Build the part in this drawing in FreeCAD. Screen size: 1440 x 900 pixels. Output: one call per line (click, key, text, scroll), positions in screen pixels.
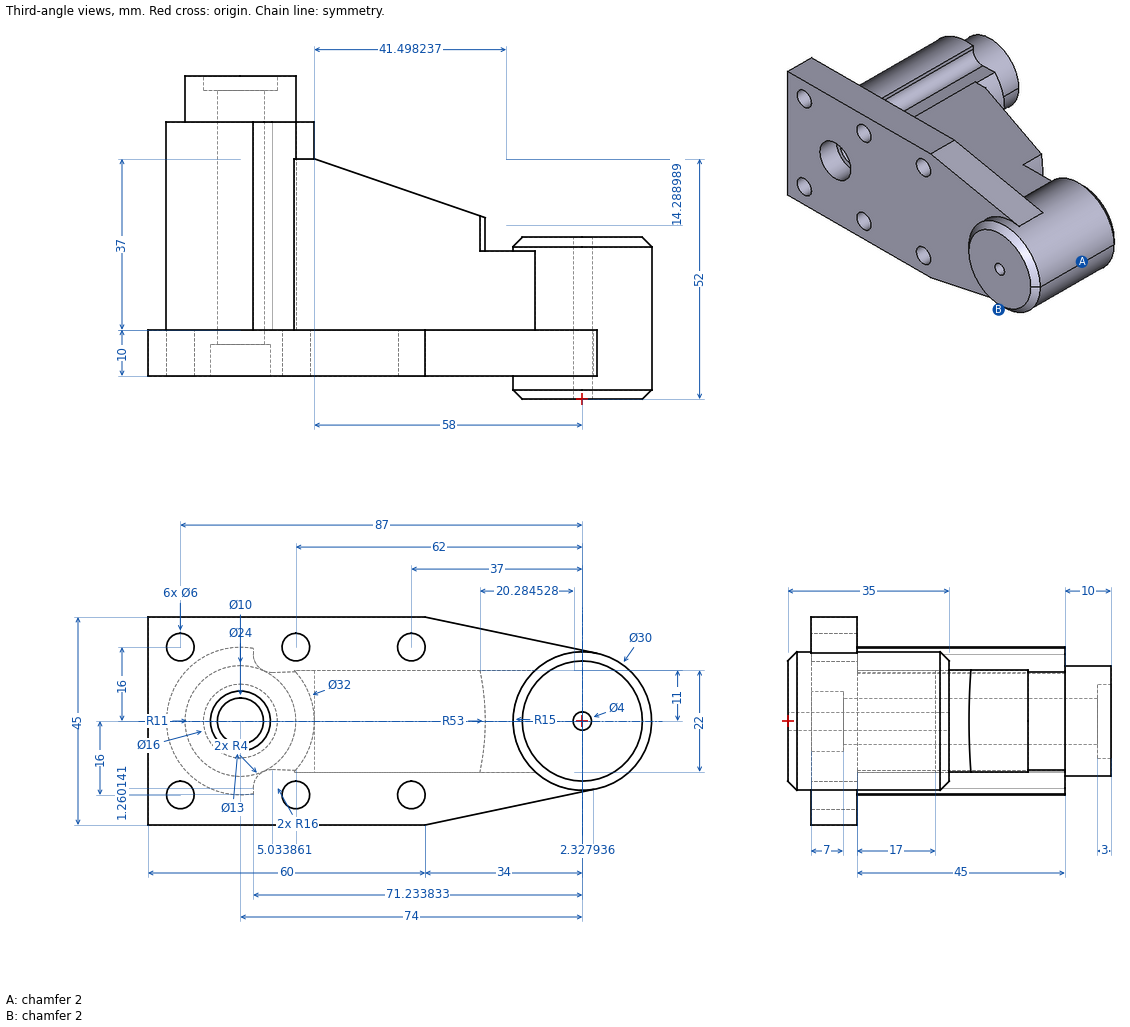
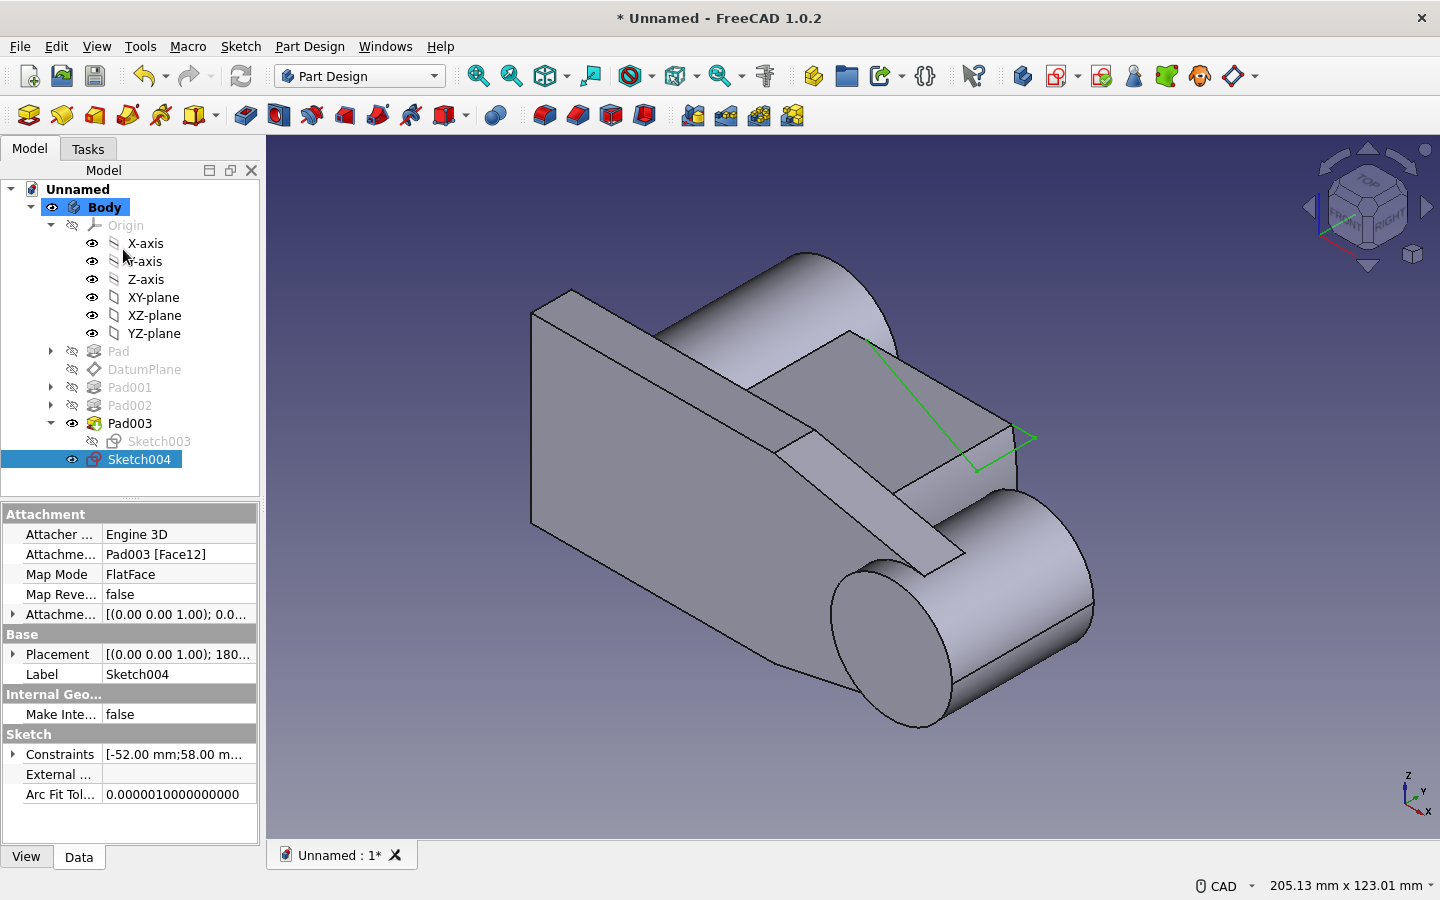
click(246, 116)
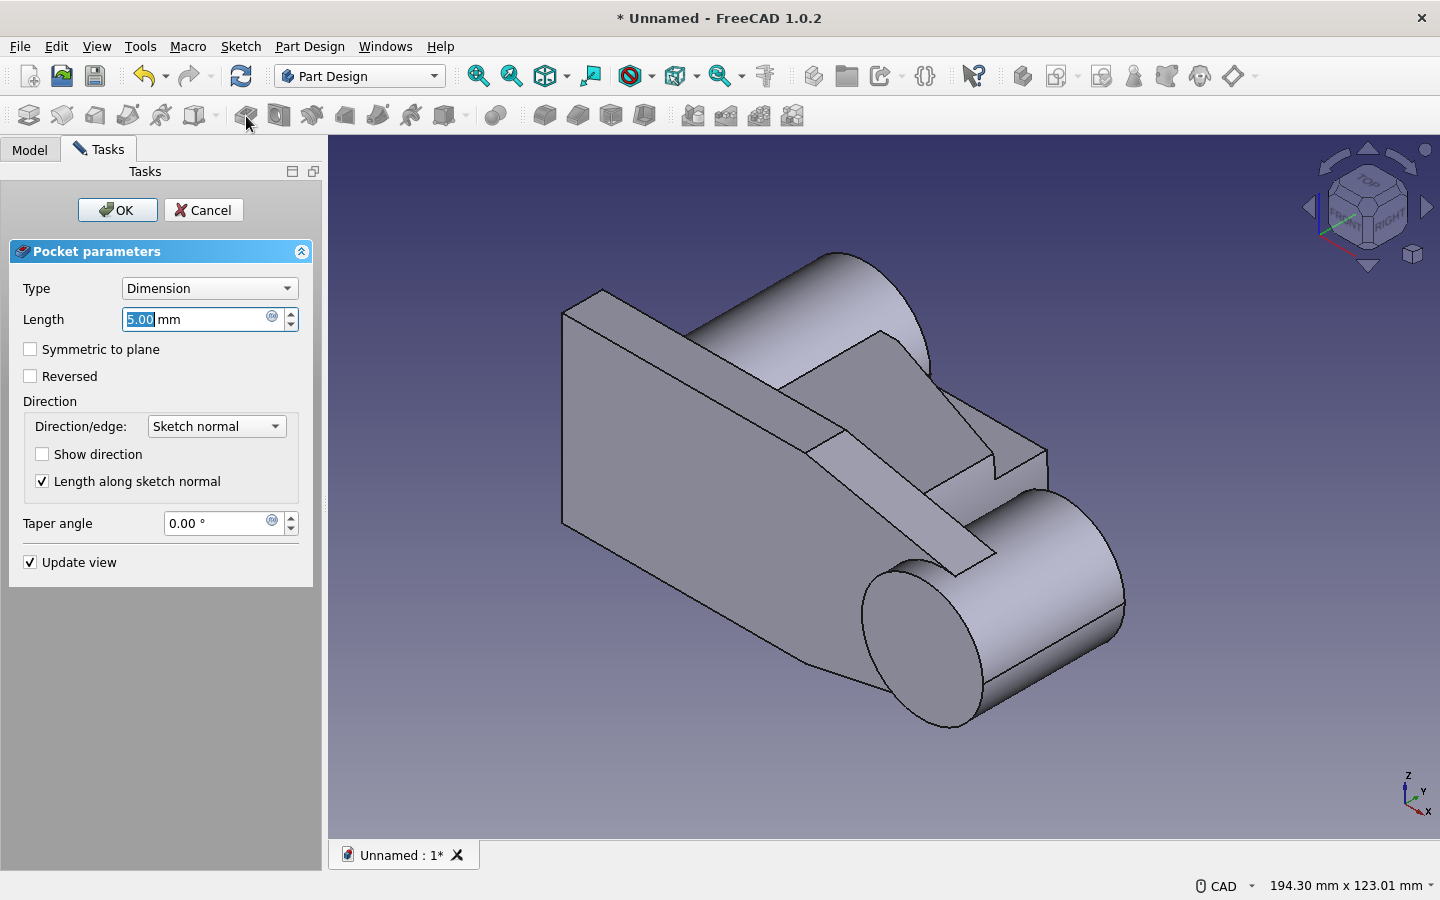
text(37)
key(Tab)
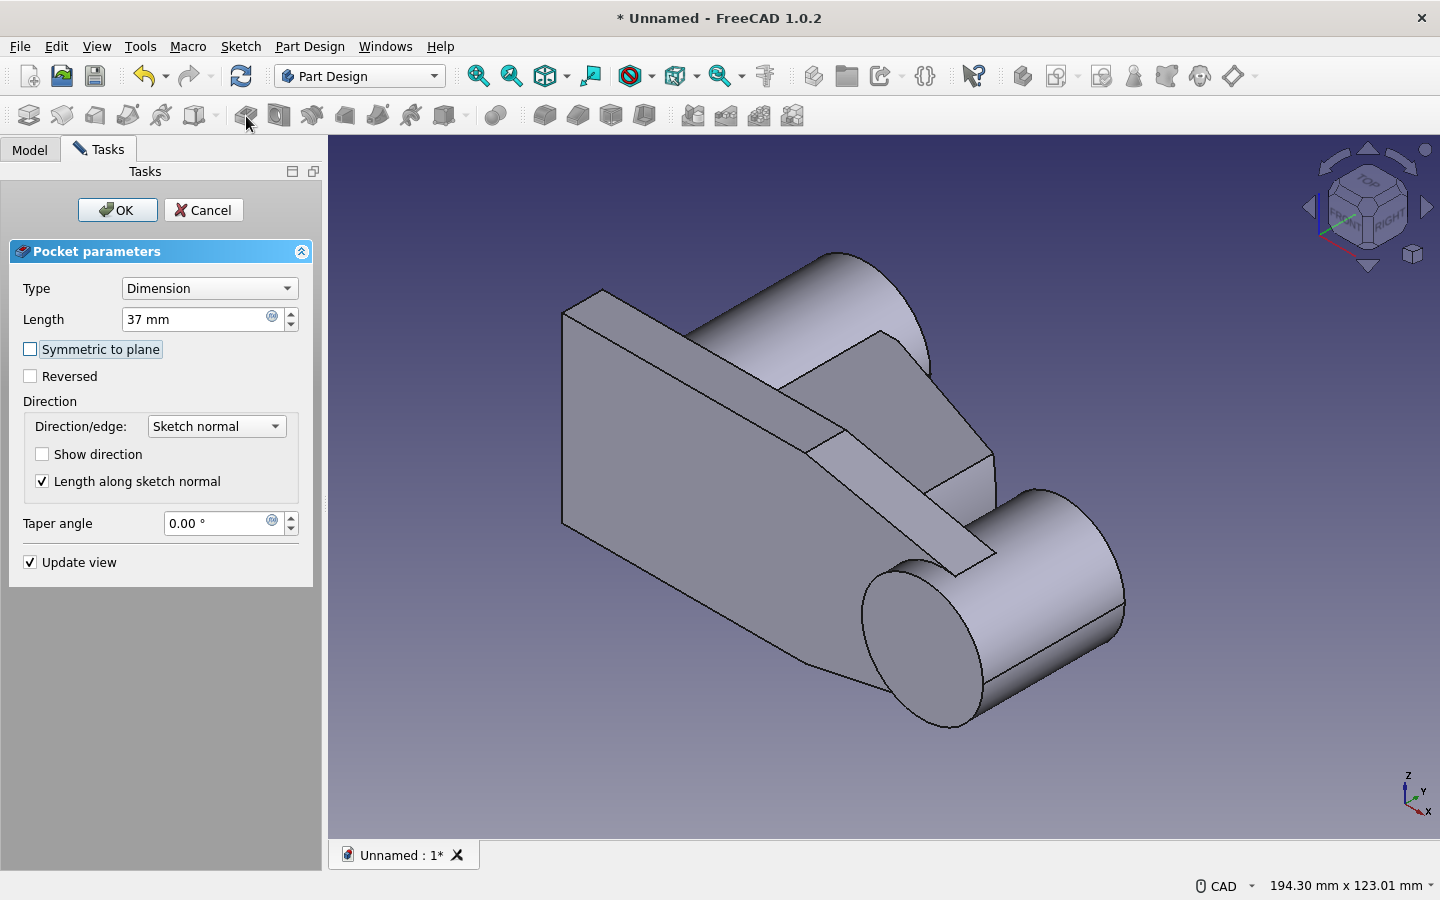
click(118, 210)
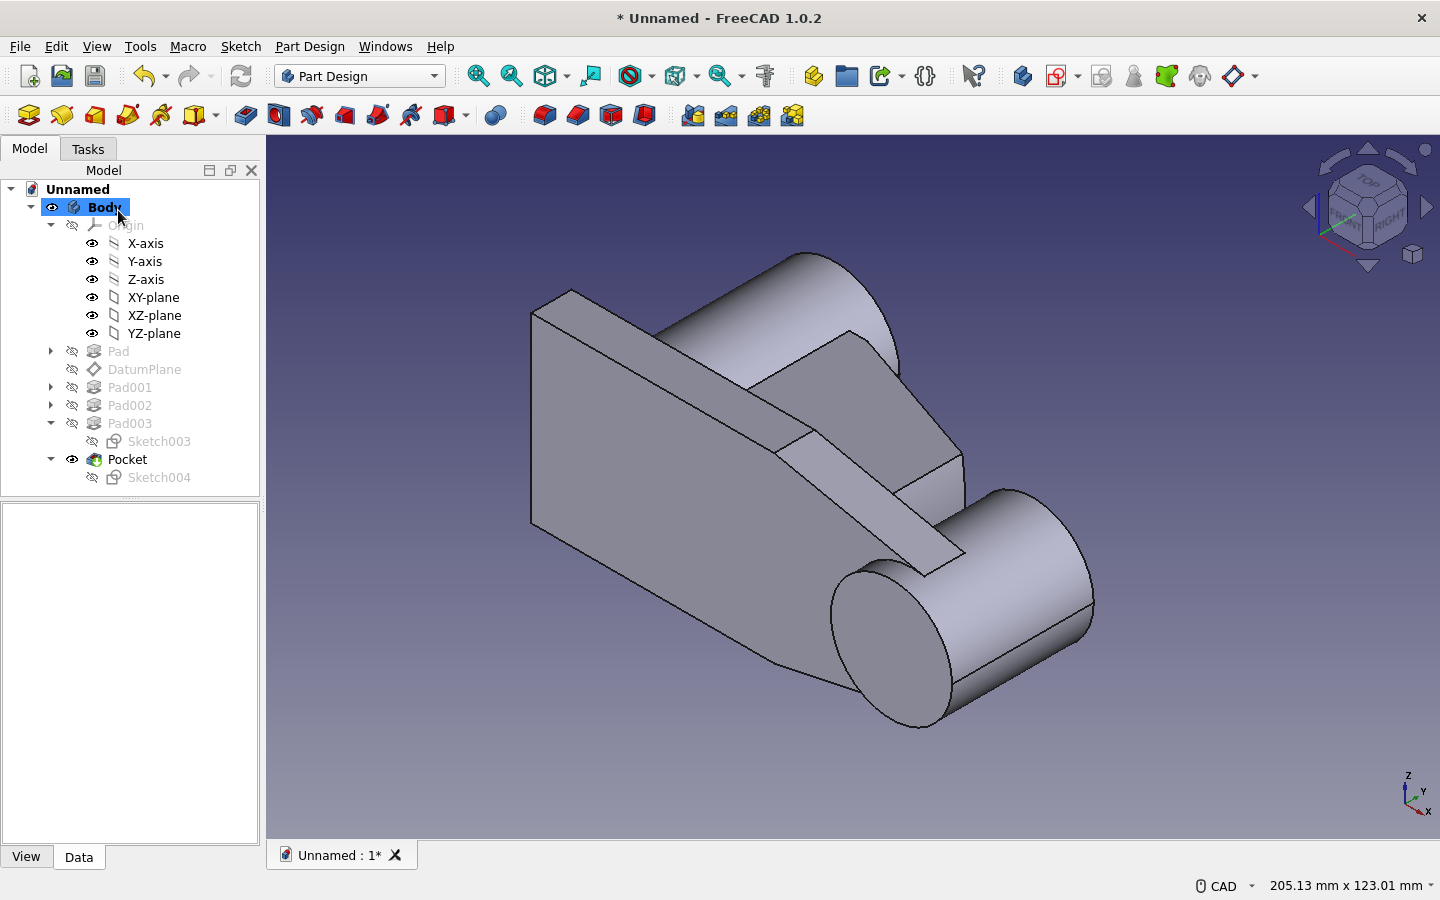
key(4)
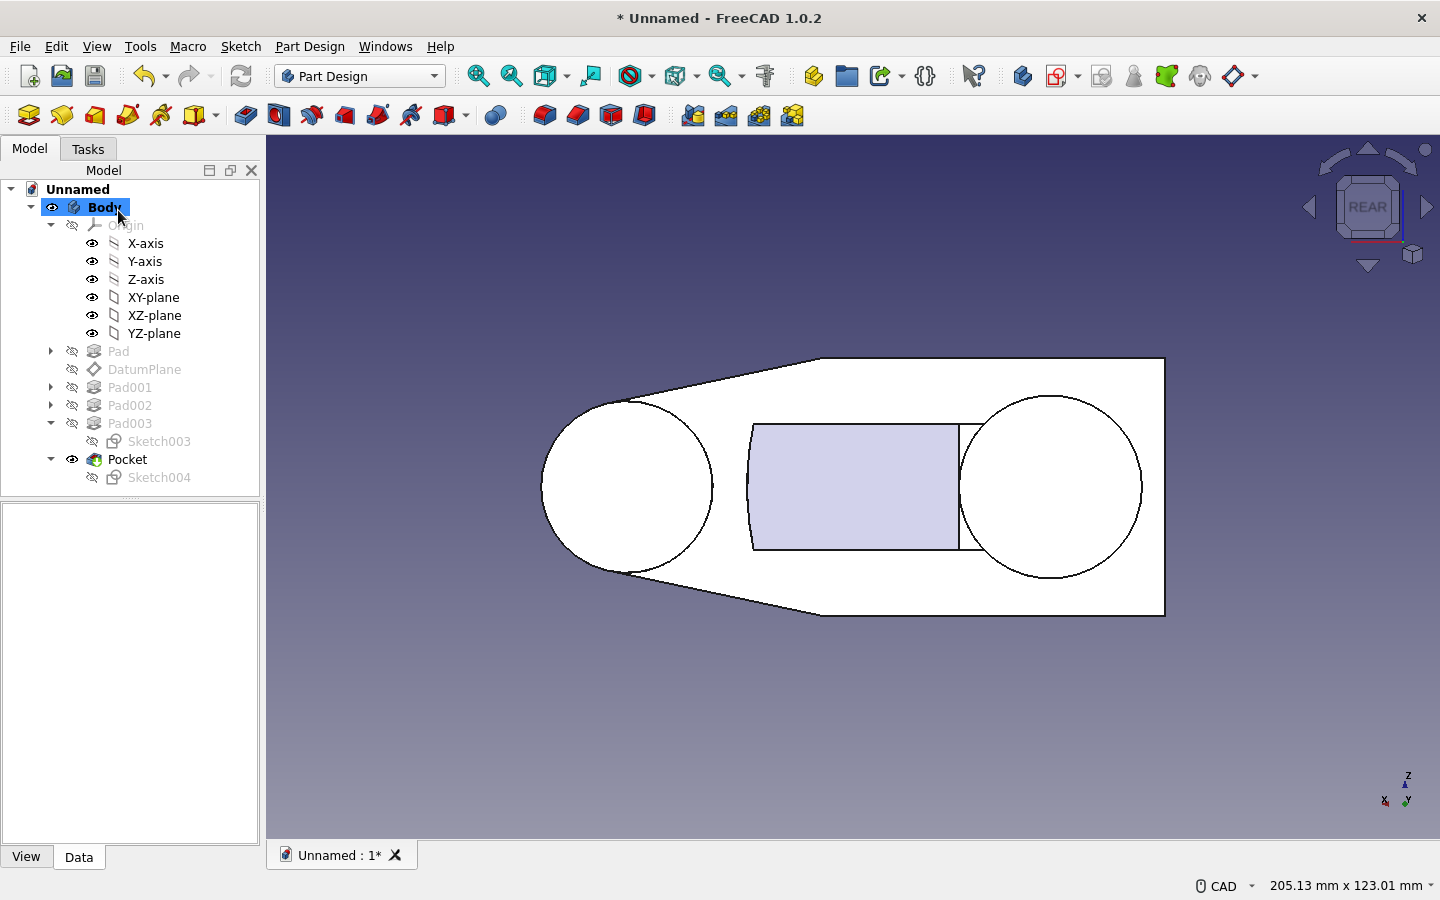
click(728, 560)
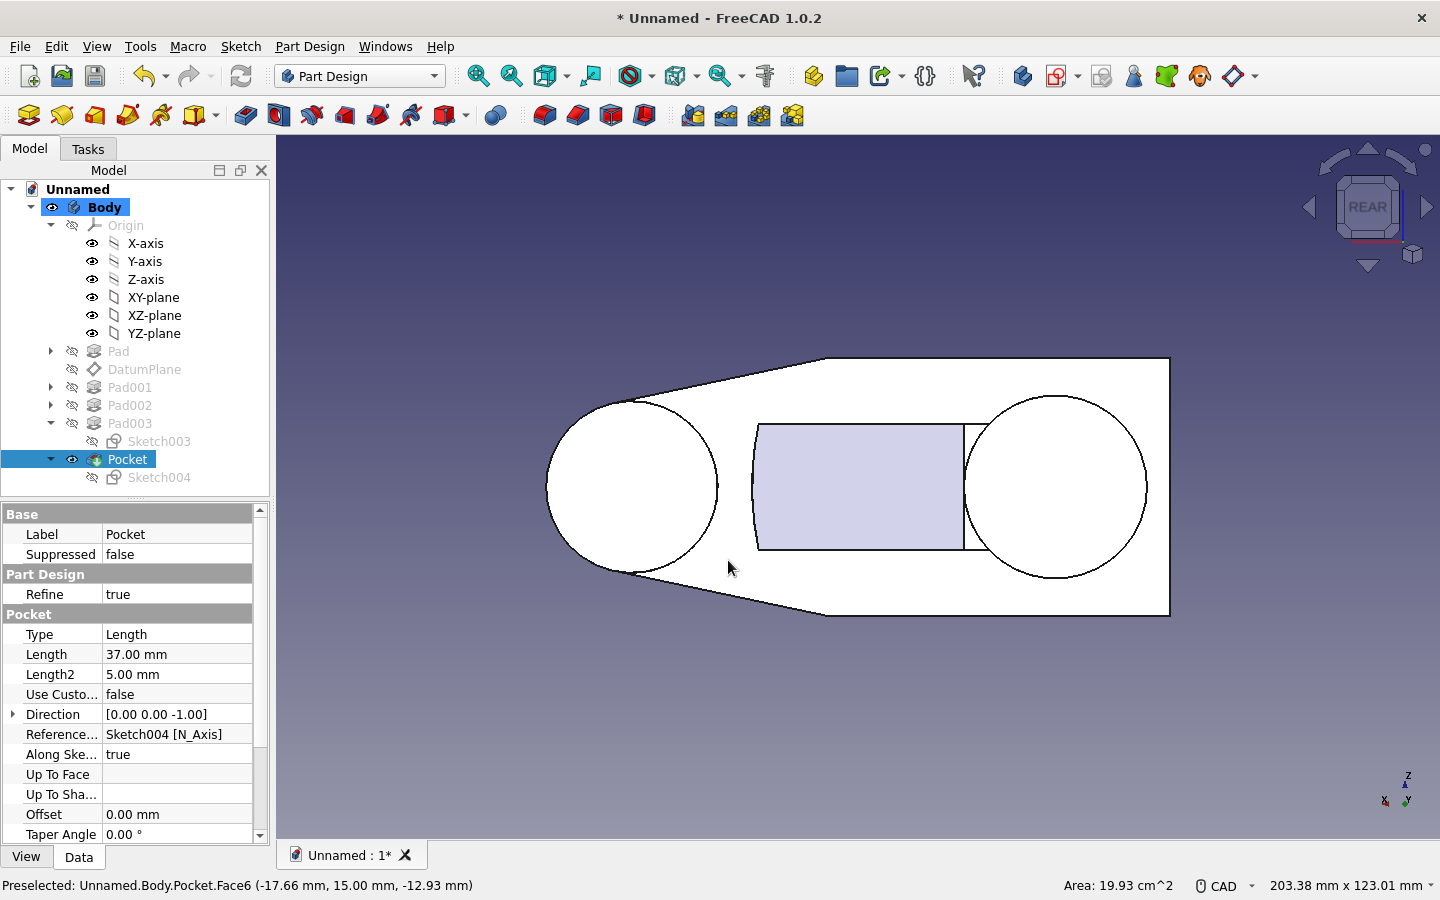
click(1056, 76)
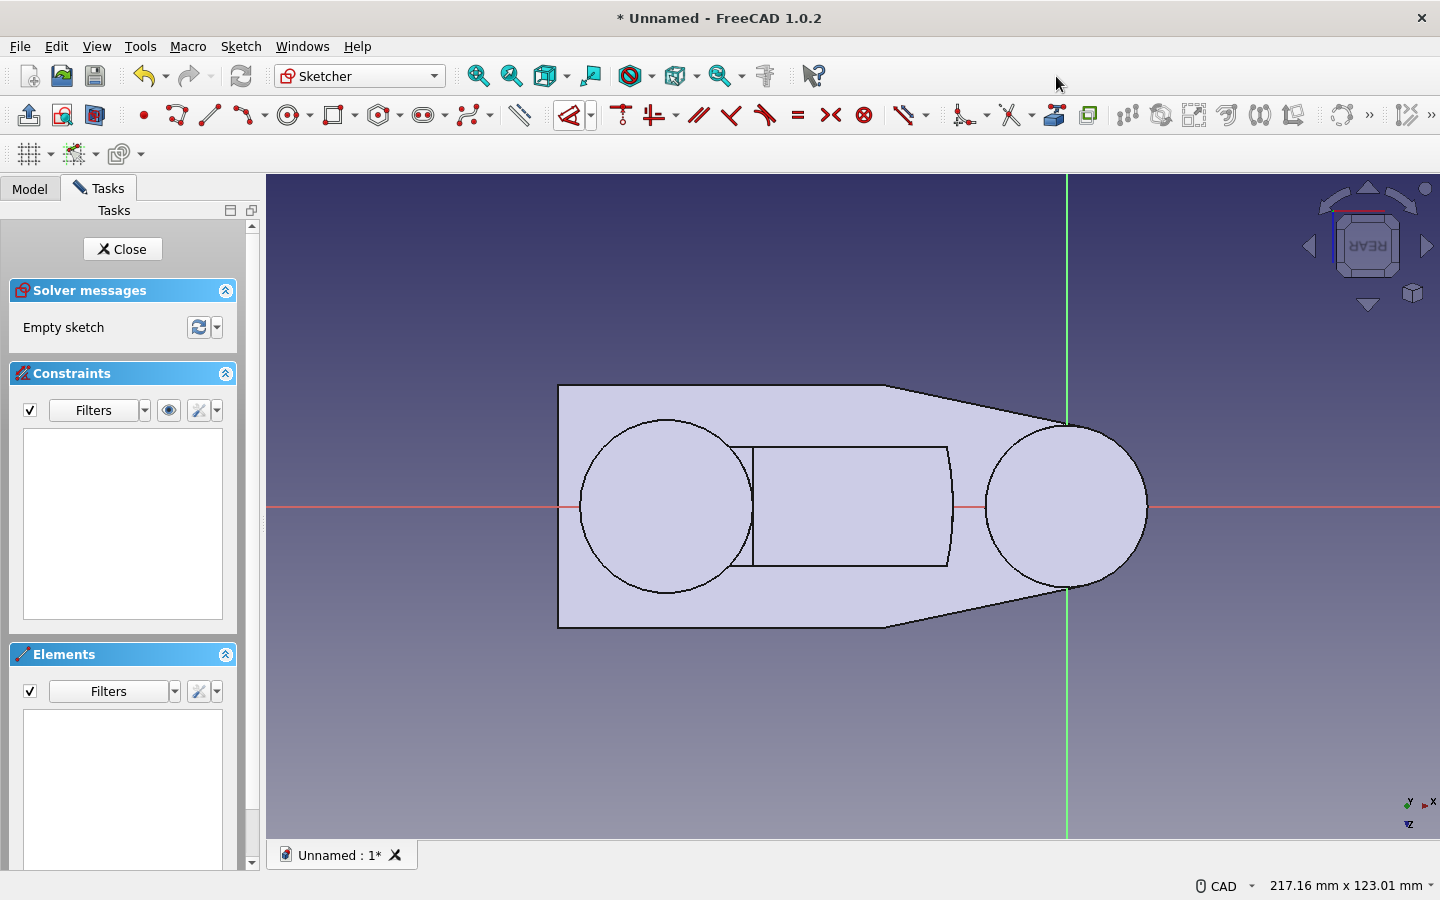
click(95, 116)